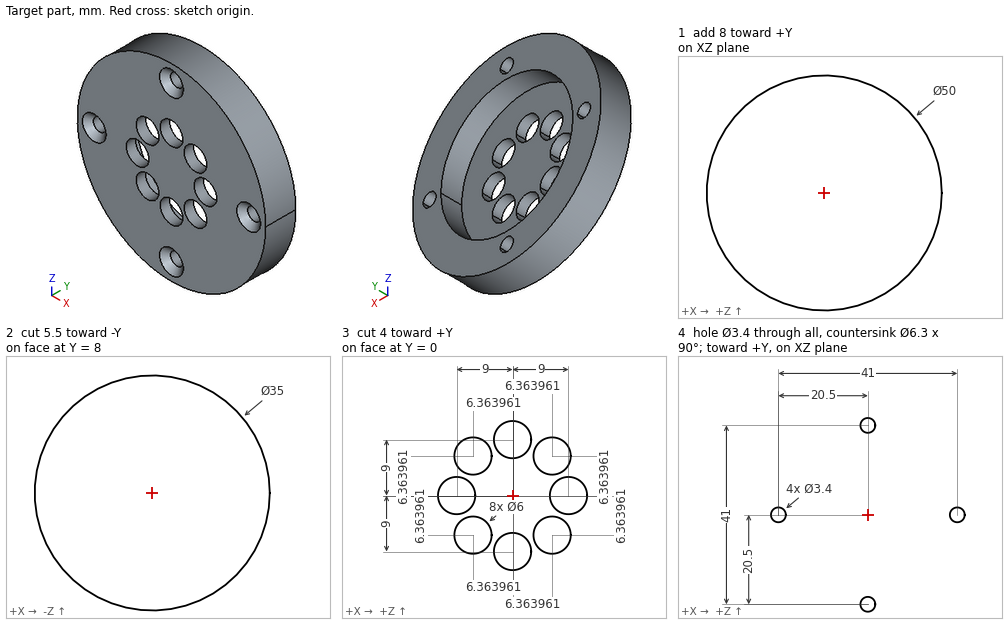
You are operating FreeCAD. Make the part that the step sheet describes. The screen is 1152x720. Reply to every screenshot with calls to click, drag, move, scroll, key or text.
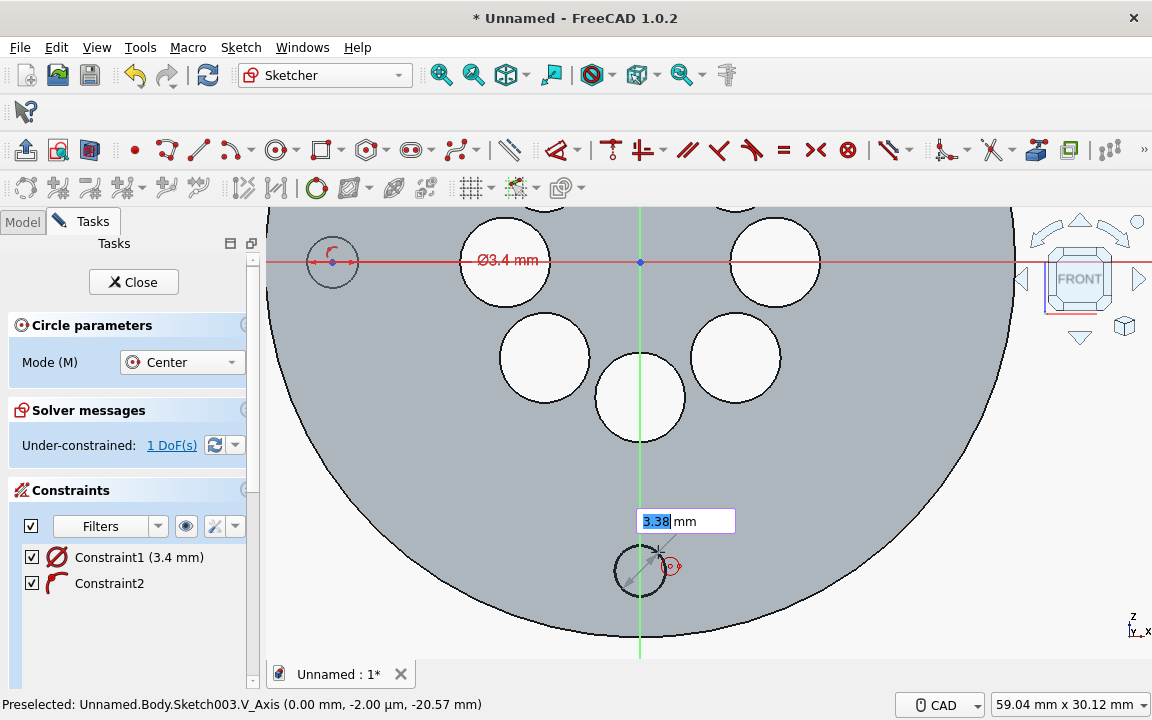
text(3.4)
key(Return)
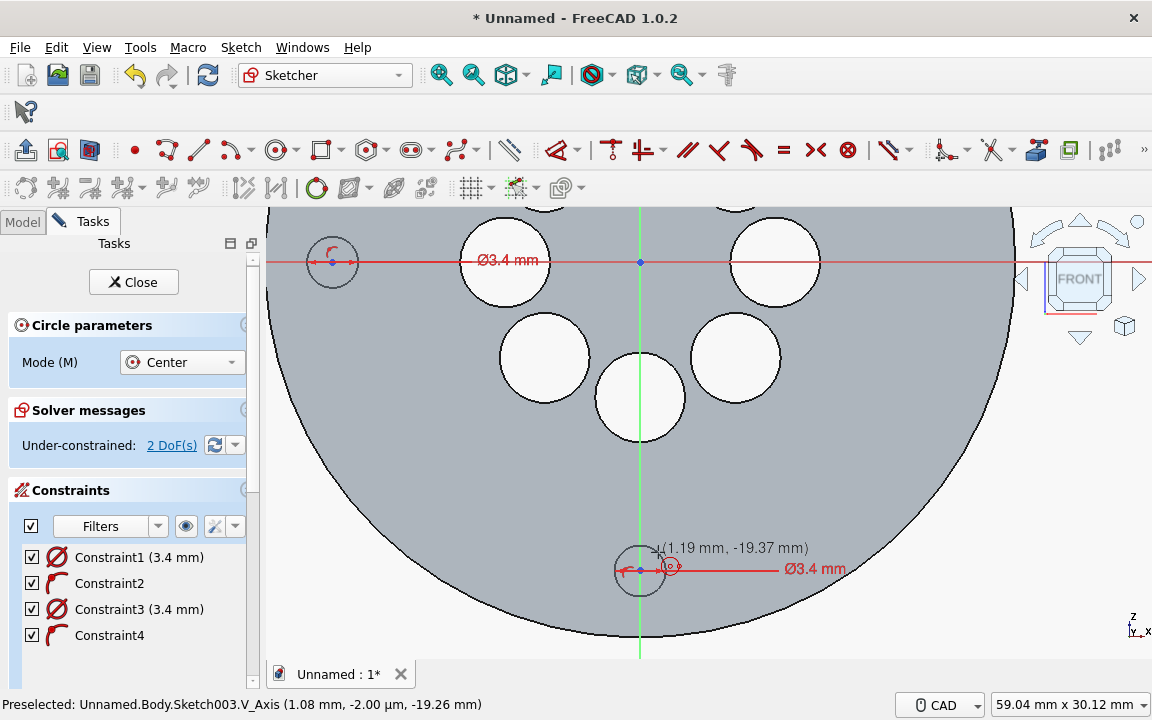
click(948, 262)
move(966, 244)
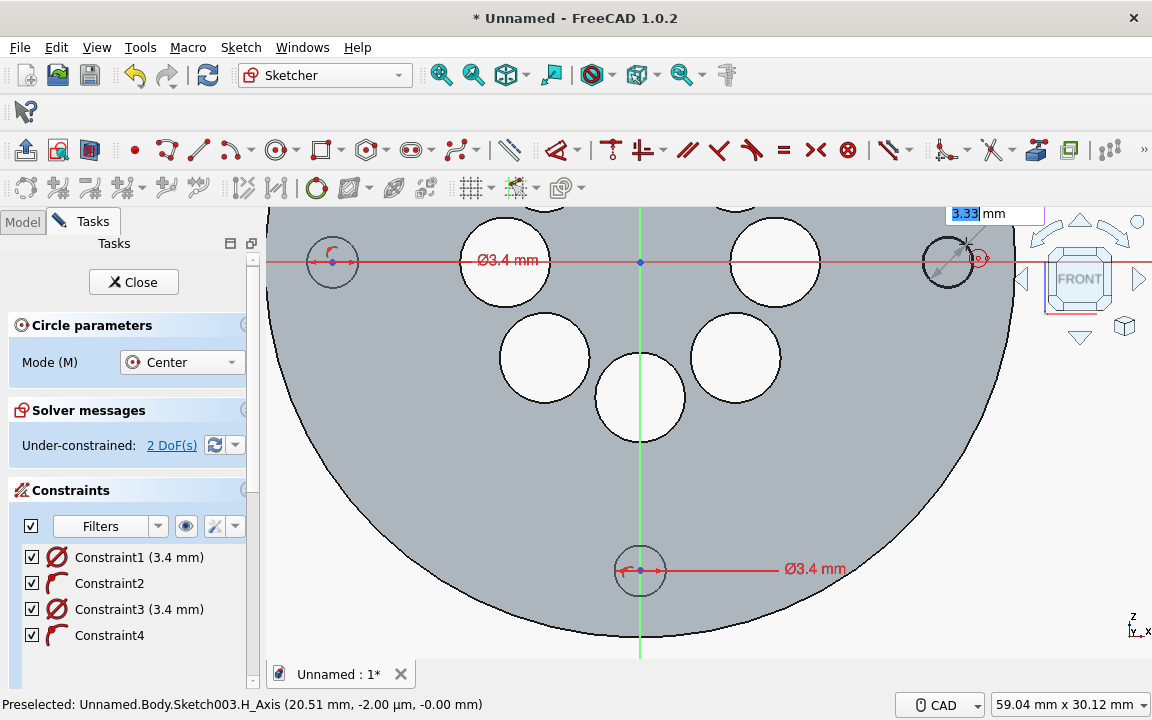
text(3.4)
key(Return)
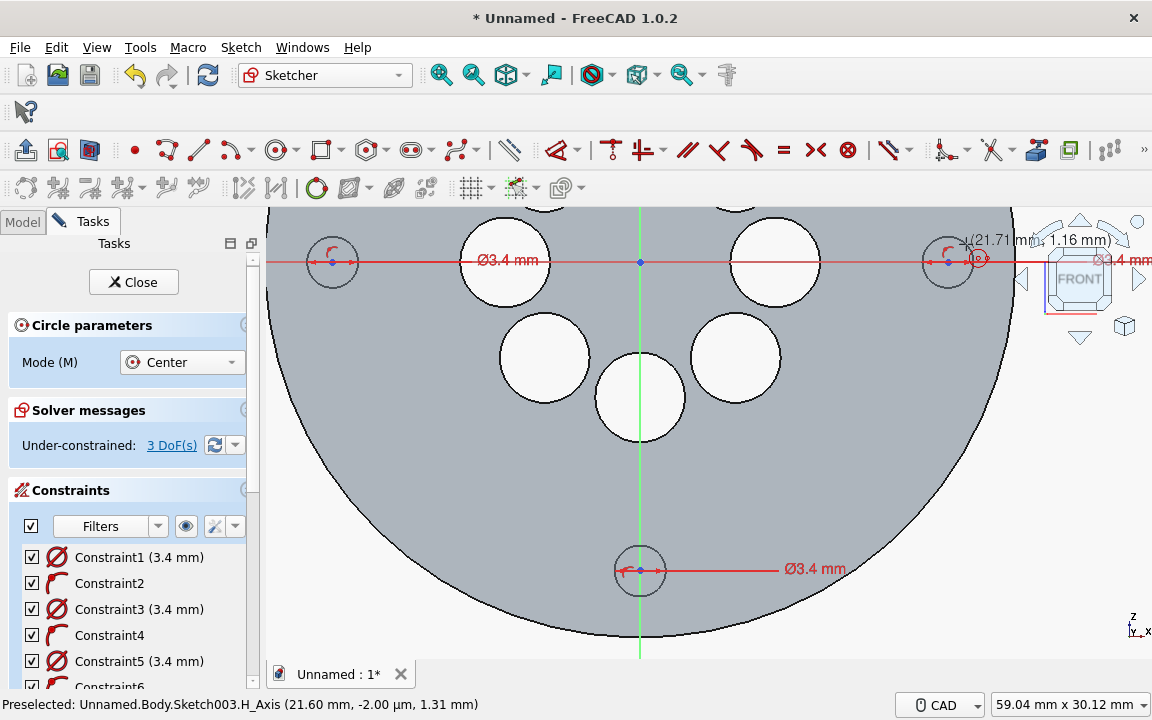
scroll(641, 572, down, 4)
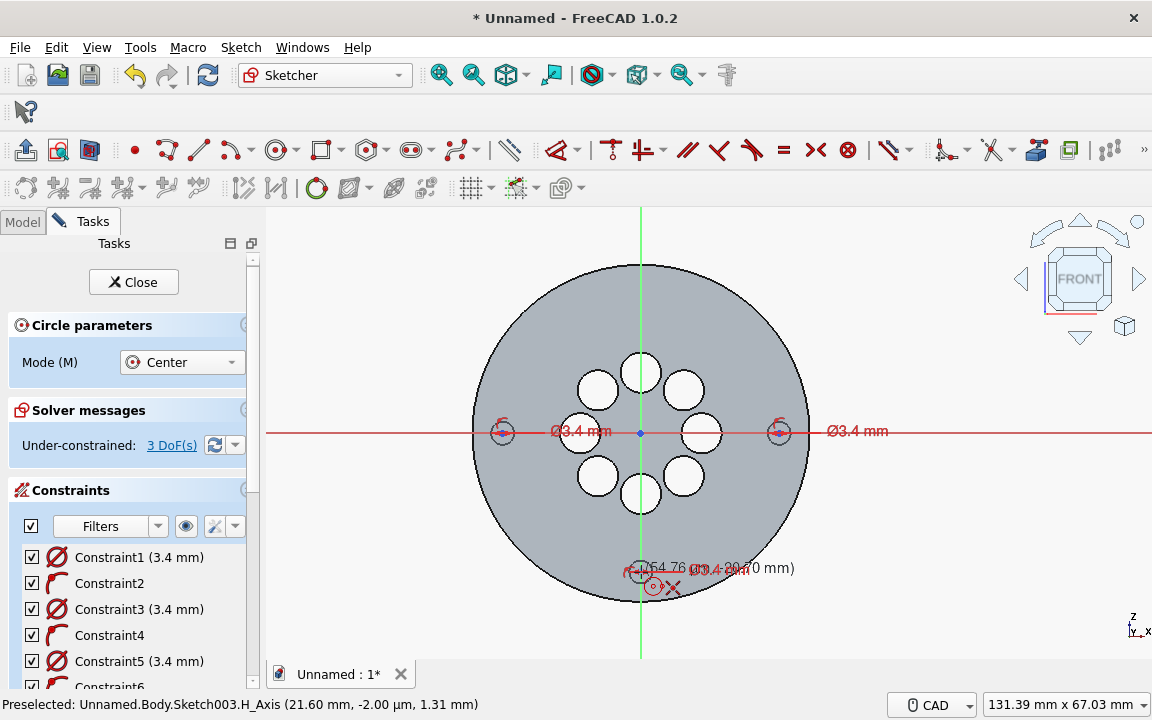
scroll(641, 295, up, 4)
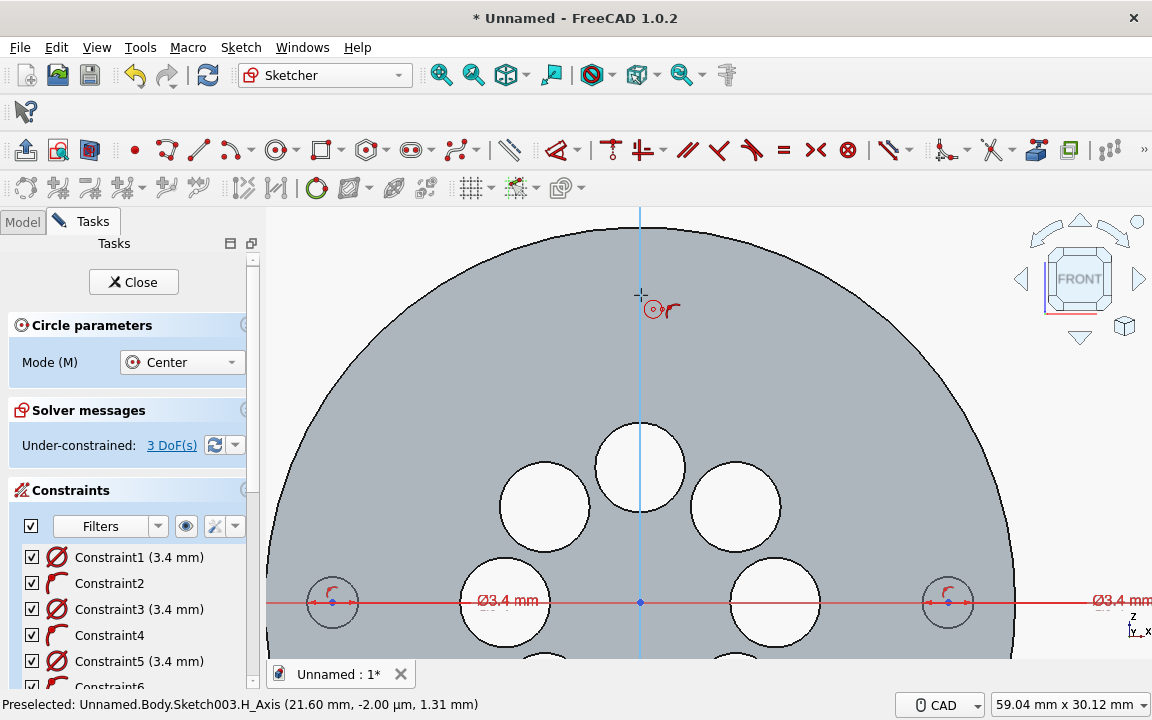
click(640, 295)
move(658, 277)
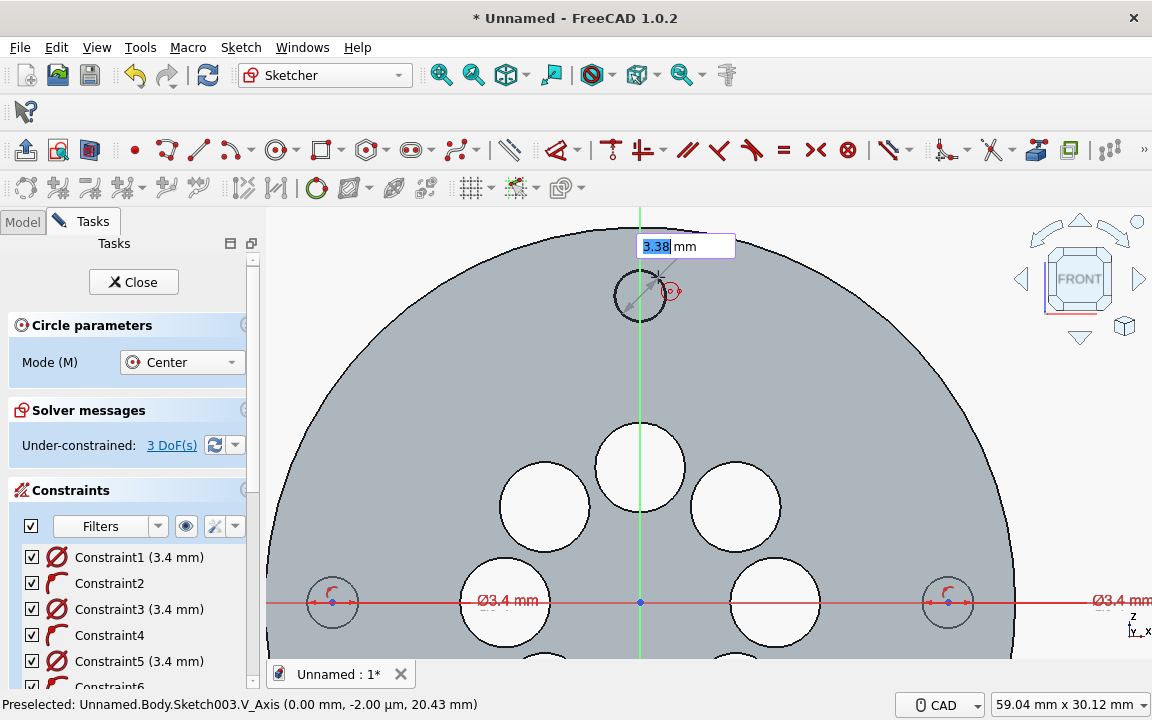
text(3.4)
key(Return)
key(Escape)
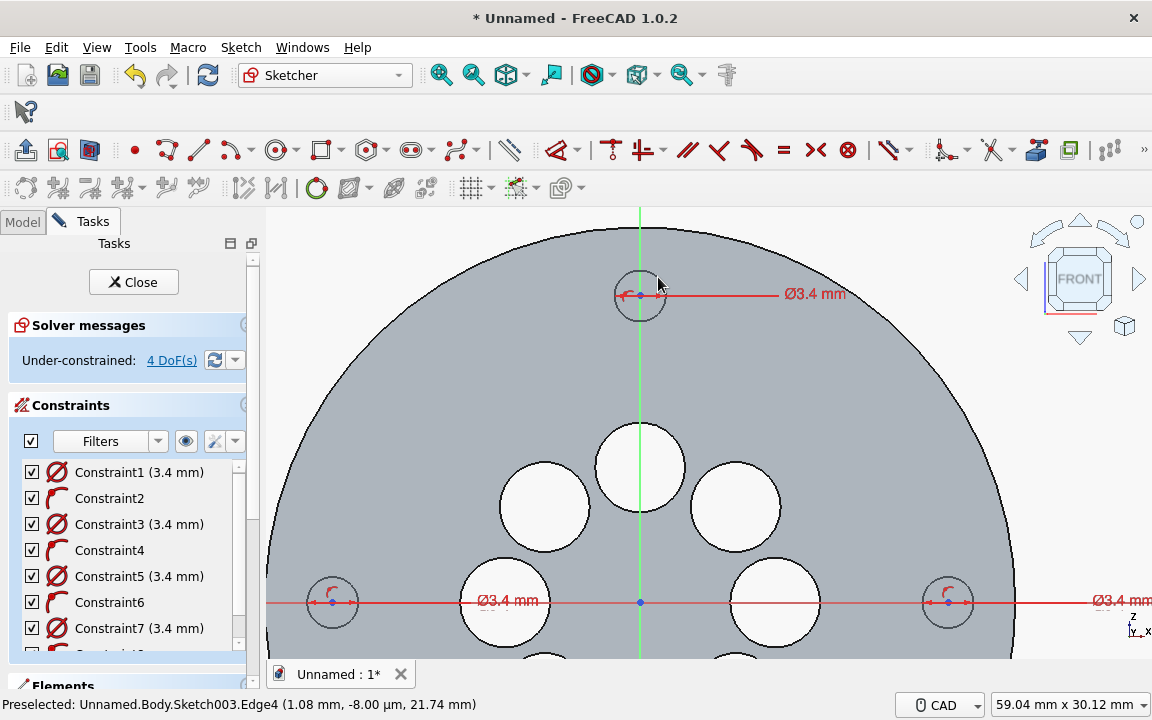
key(d)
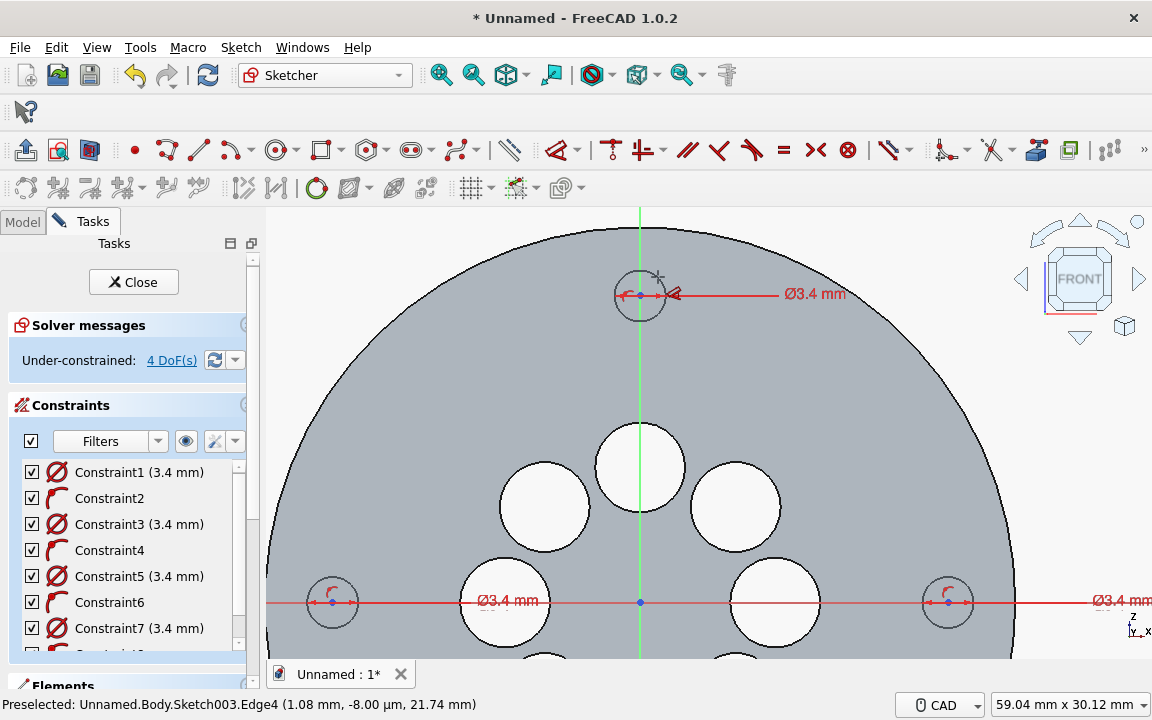
click(333, 603)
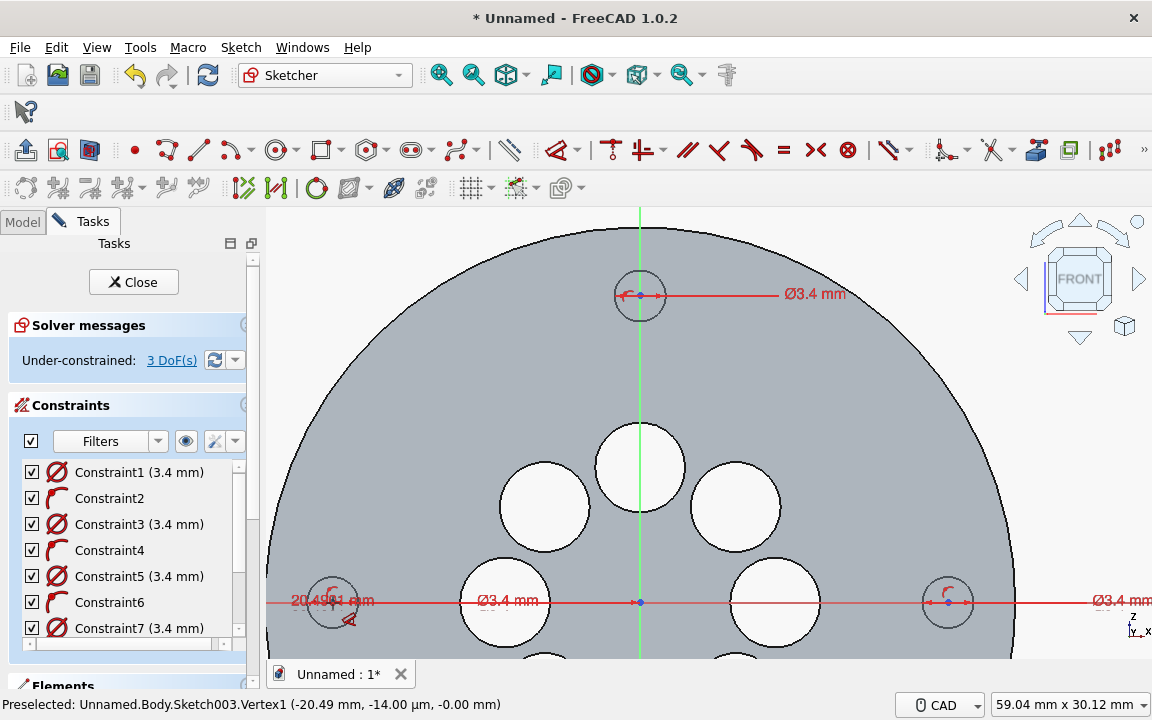
click(948, 603)
click(499, 569)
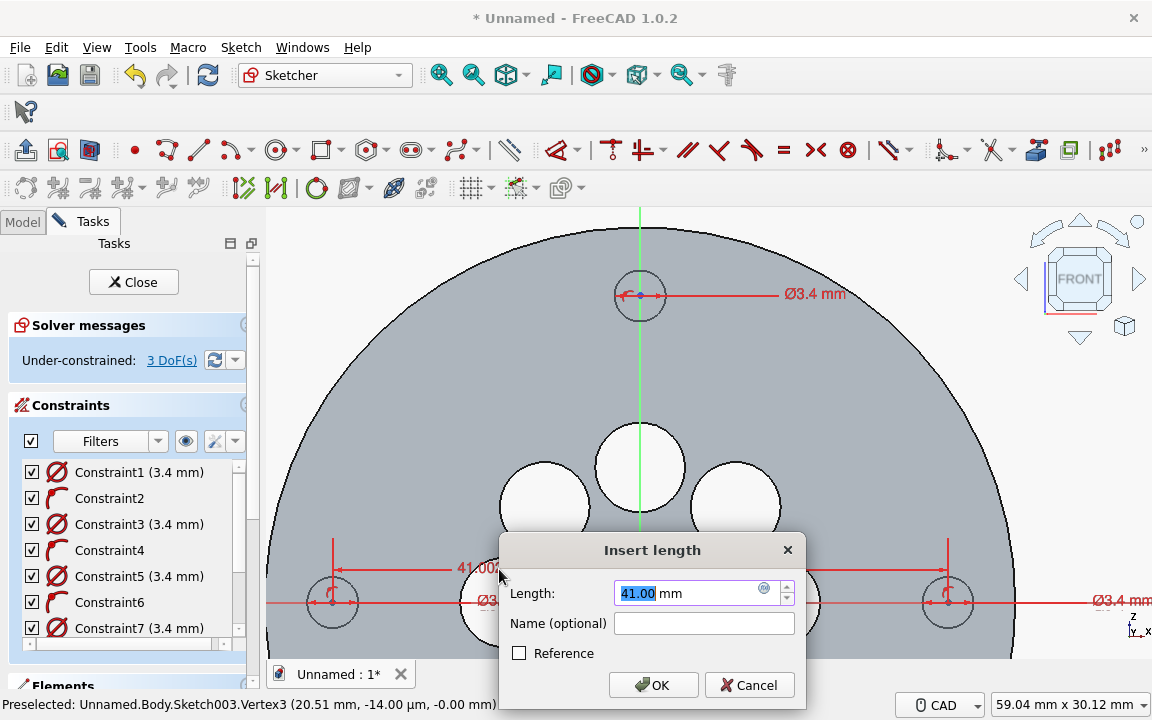
text(41)
key(Return)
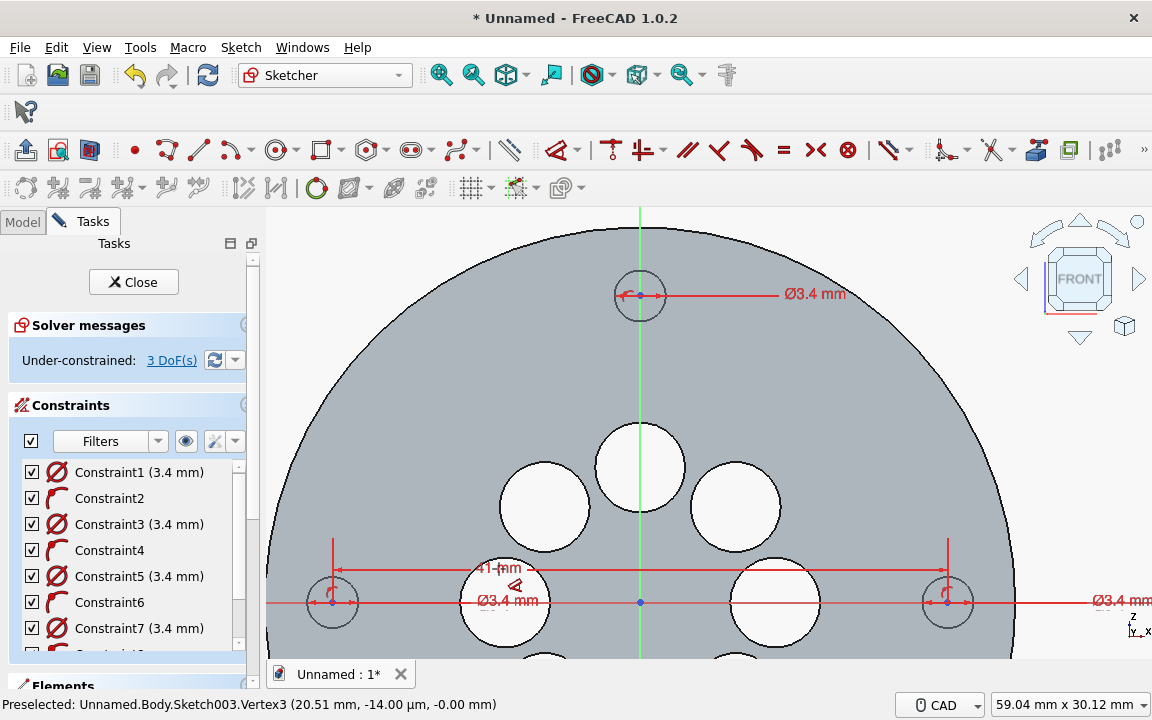
scroll(641, 295, down, 4)